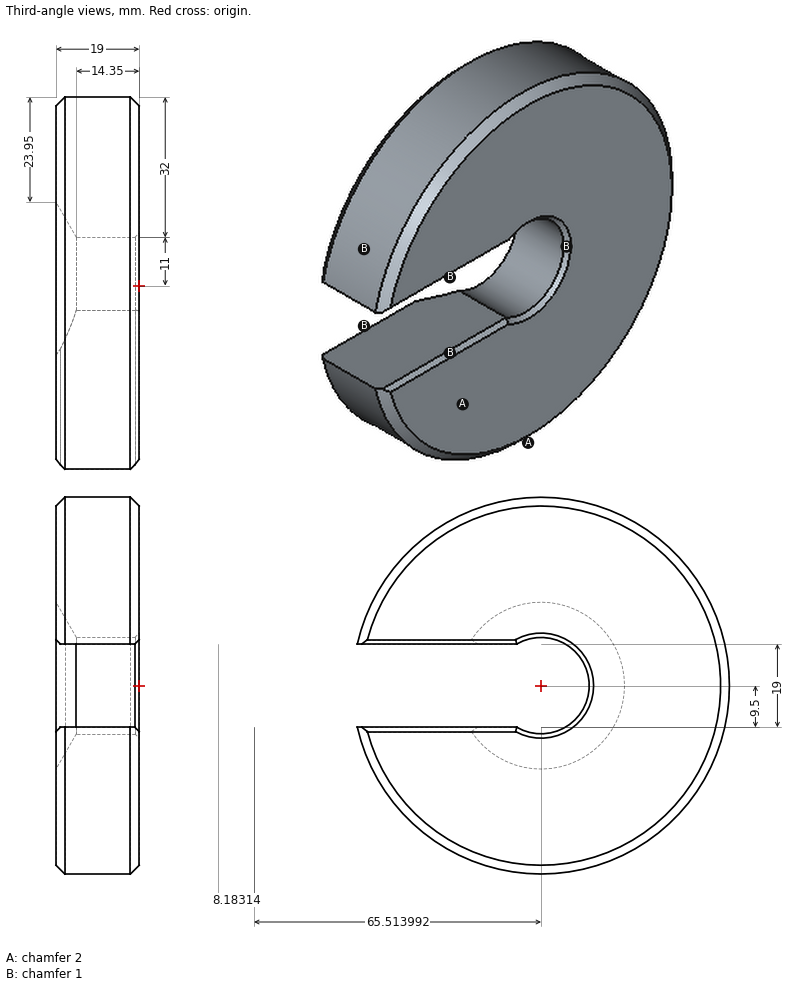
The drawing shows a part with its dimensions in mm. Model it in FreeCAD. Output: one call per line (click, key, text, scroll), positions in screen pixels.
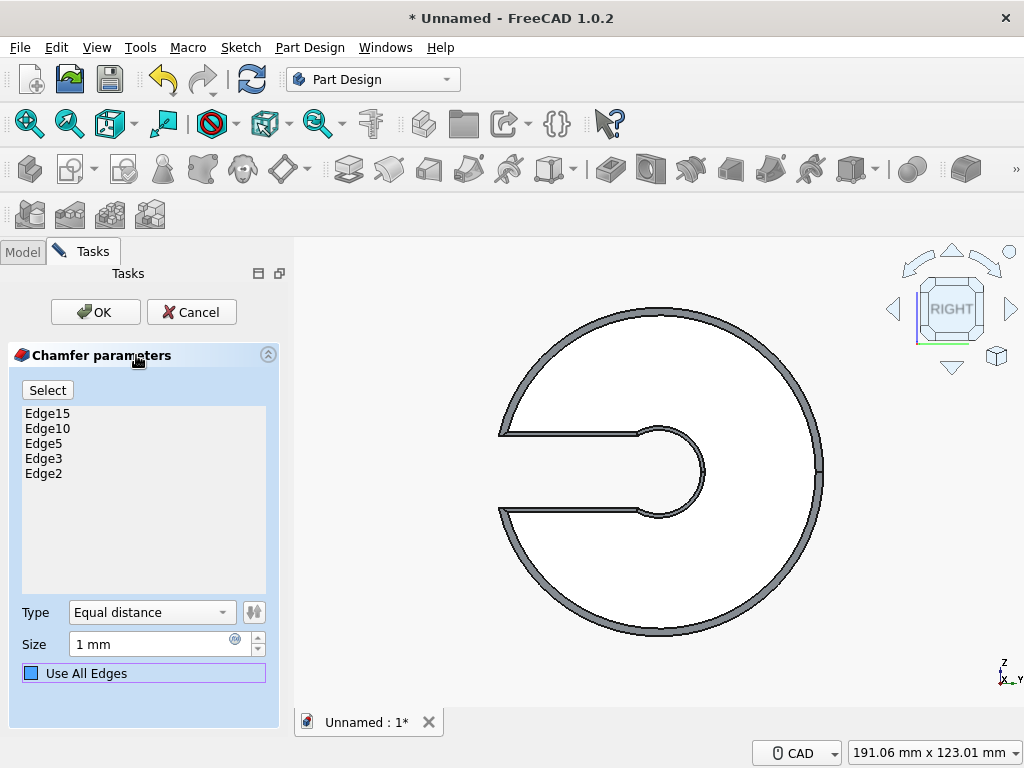
click(96, 312)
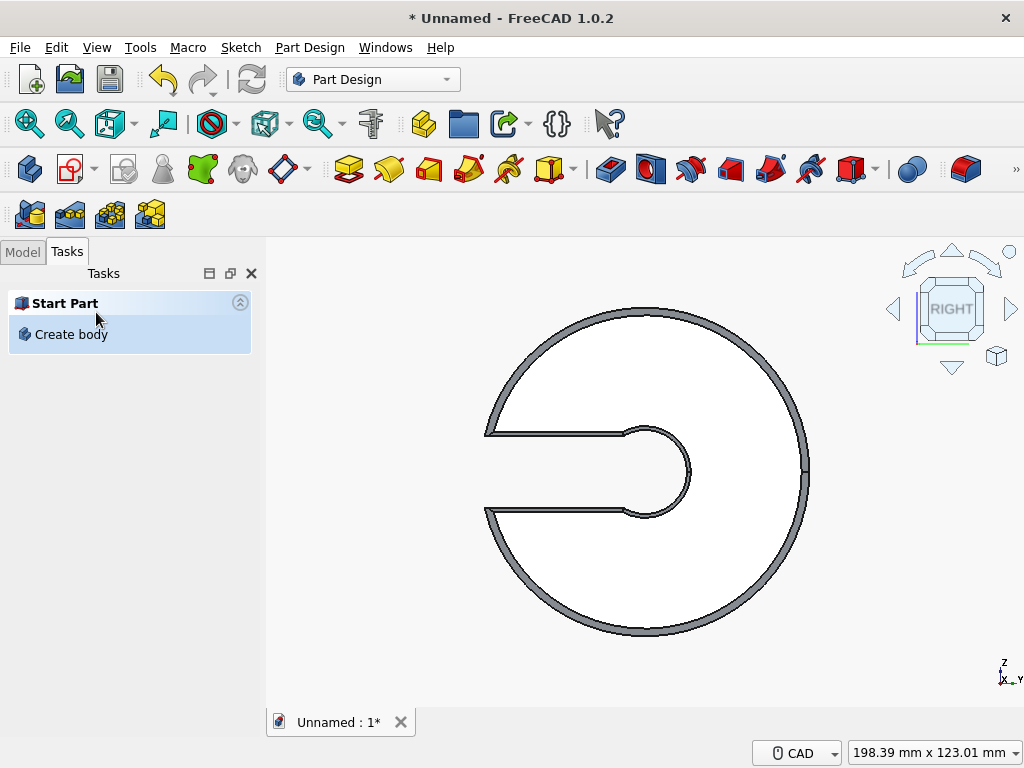
key(0)